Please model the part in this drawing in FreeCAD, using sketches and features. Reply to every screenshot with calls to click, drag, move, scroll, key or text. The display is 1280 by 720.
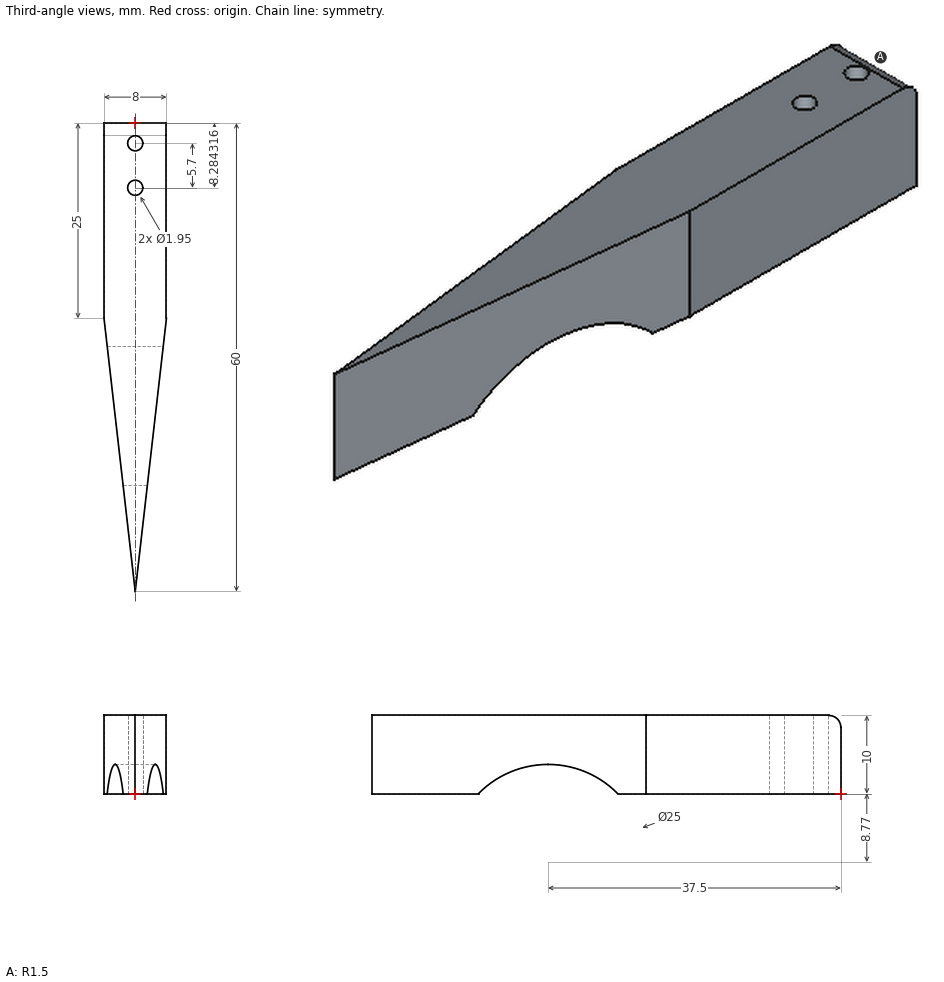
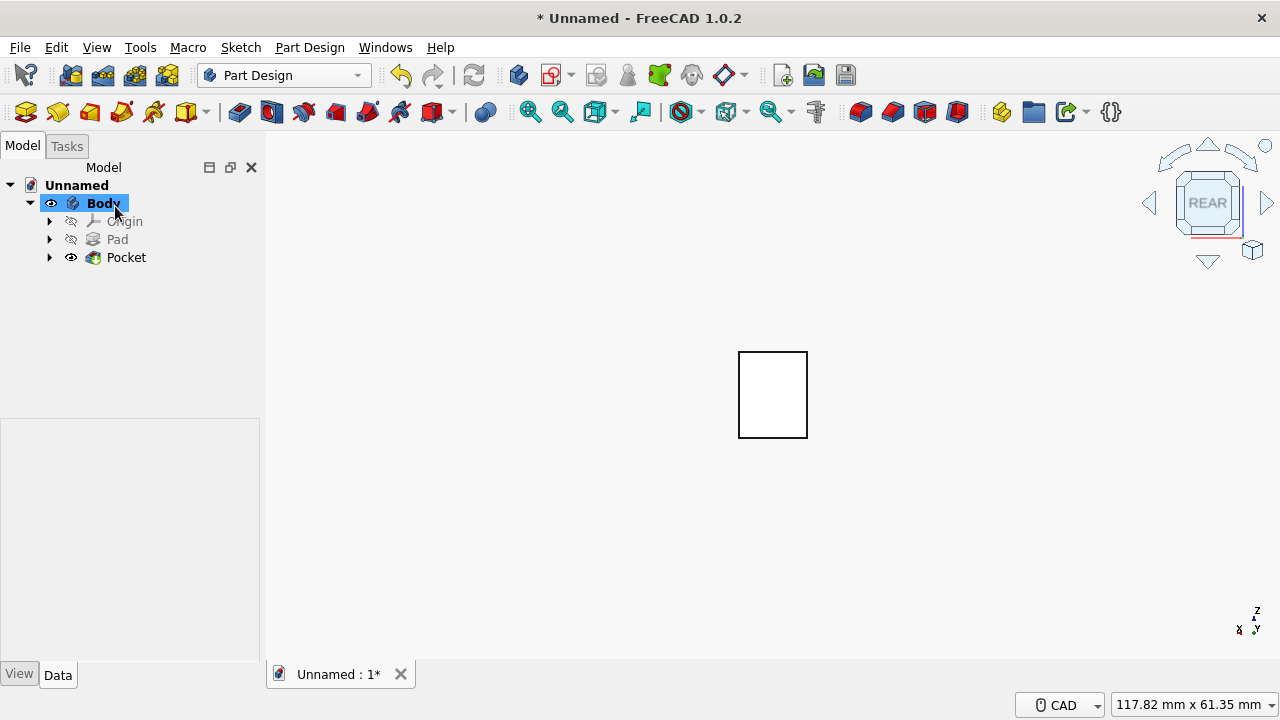
click(532, 112)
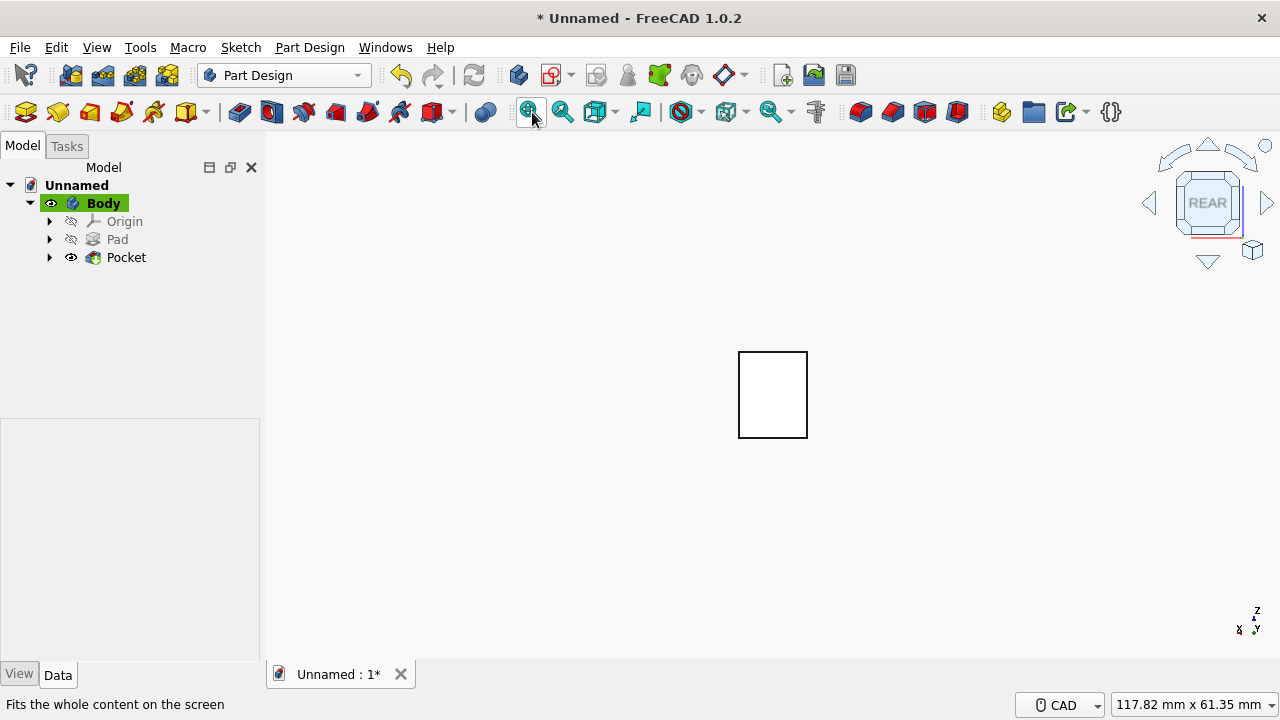
click(773, 351)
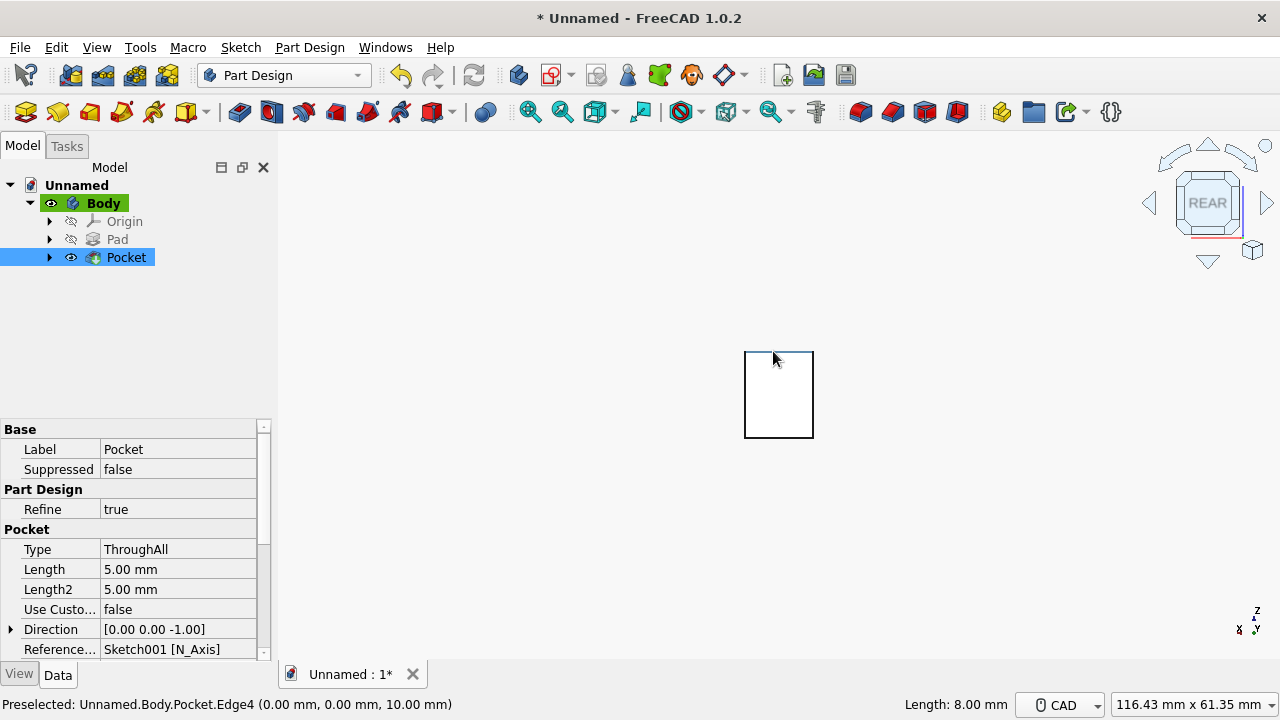
click(862, 112)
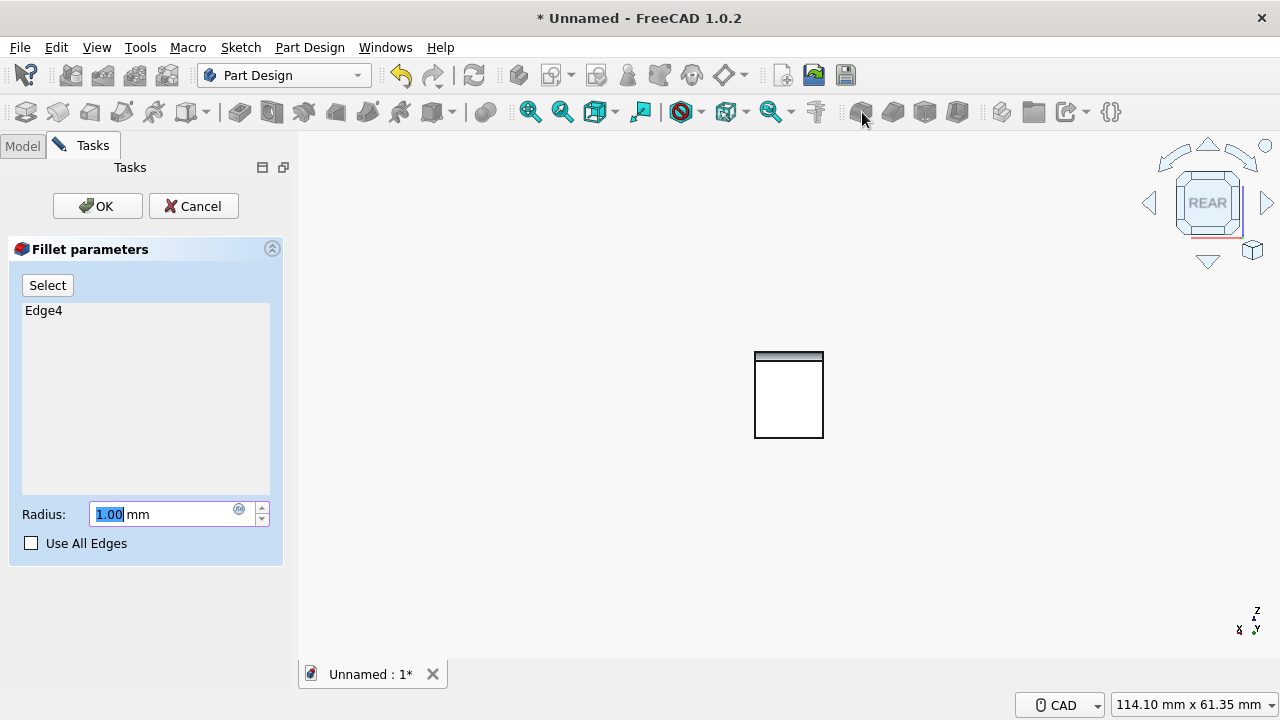
text(1.5)
key(Tab)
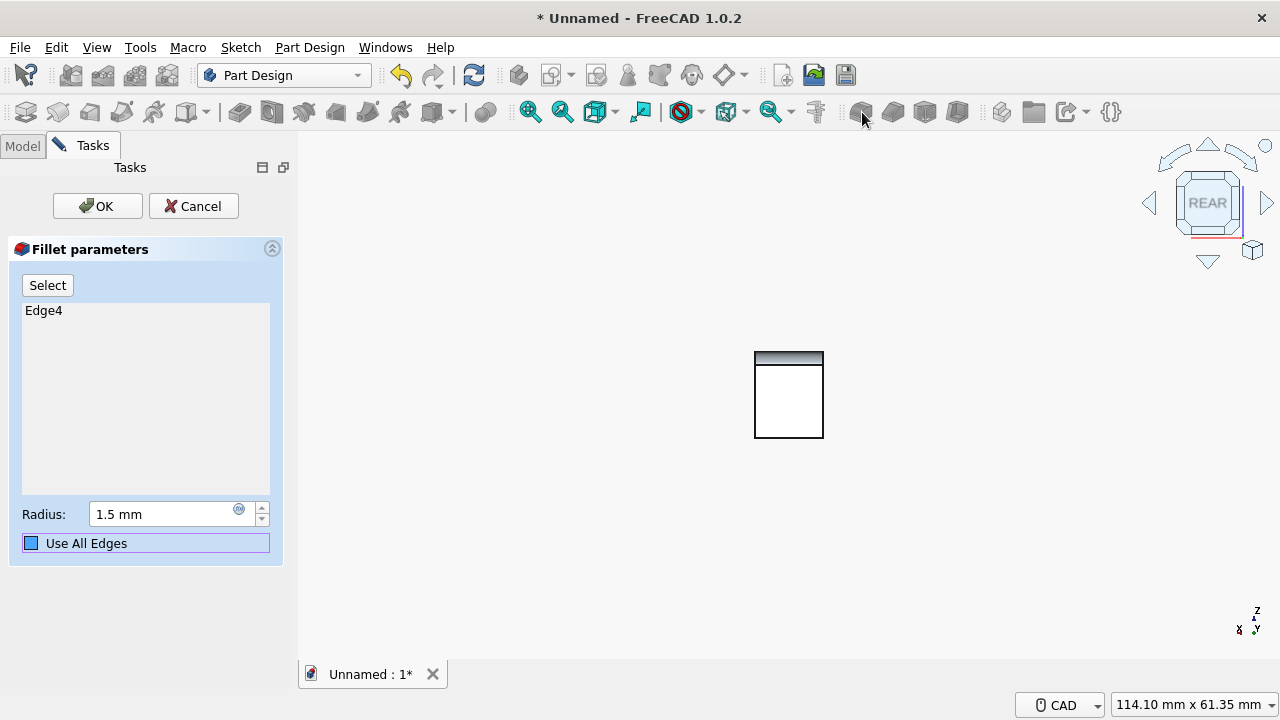
click(98, 206)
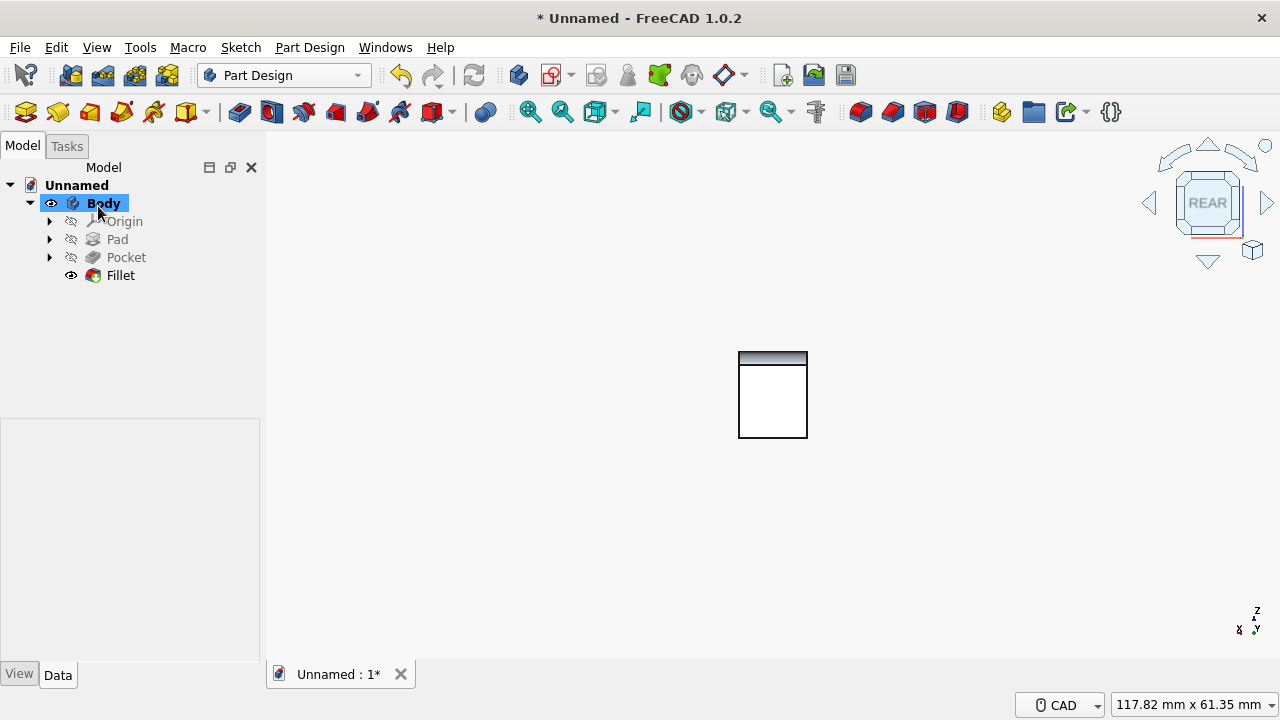
key(v)
key(f)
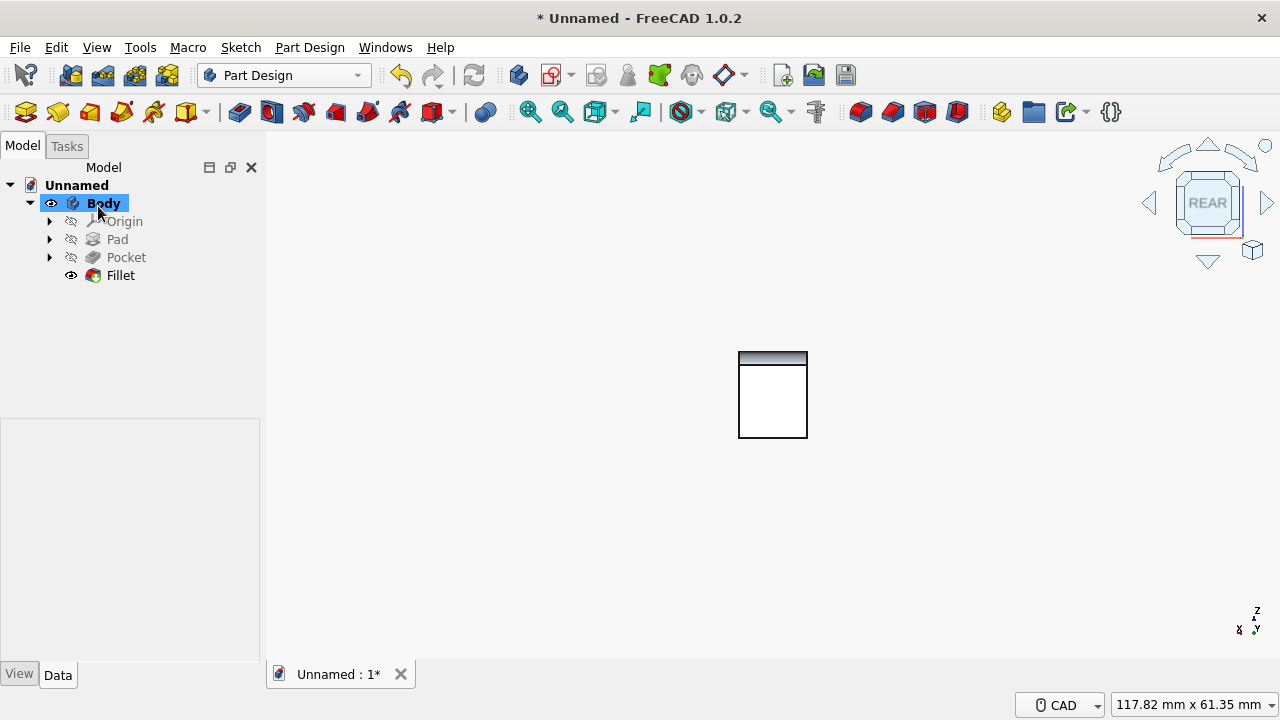
key(6)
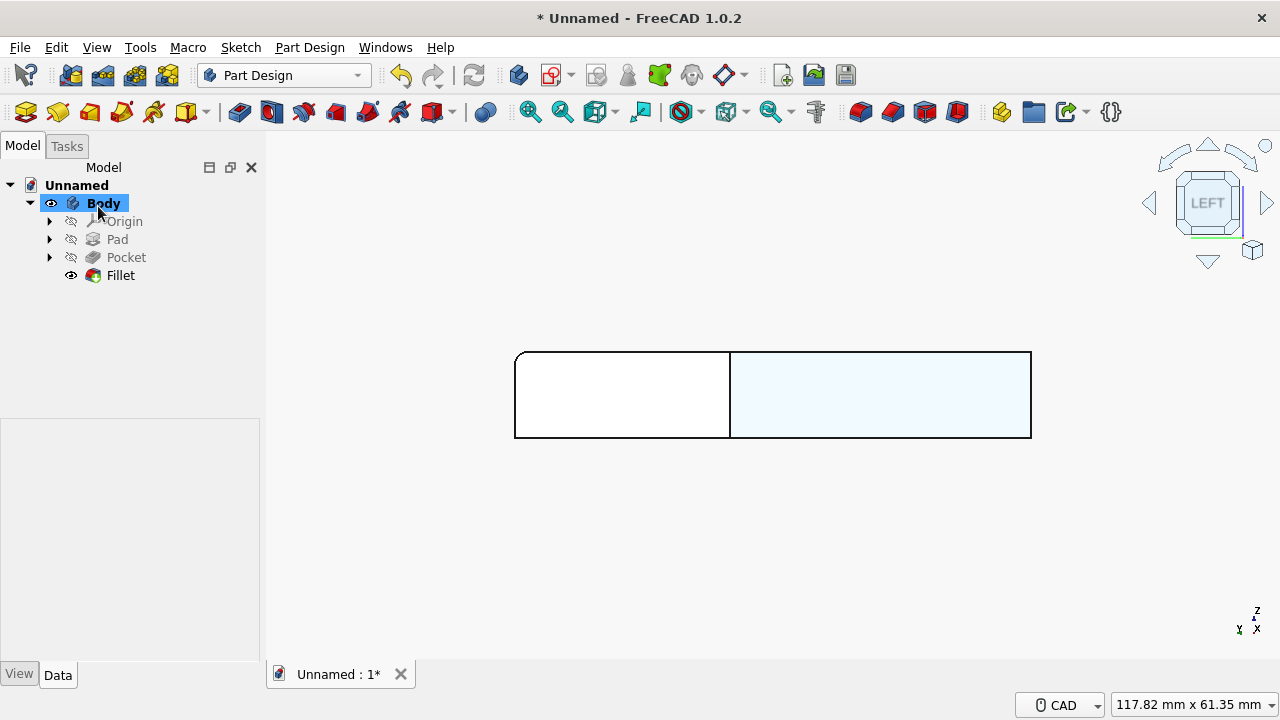
click(561, 394)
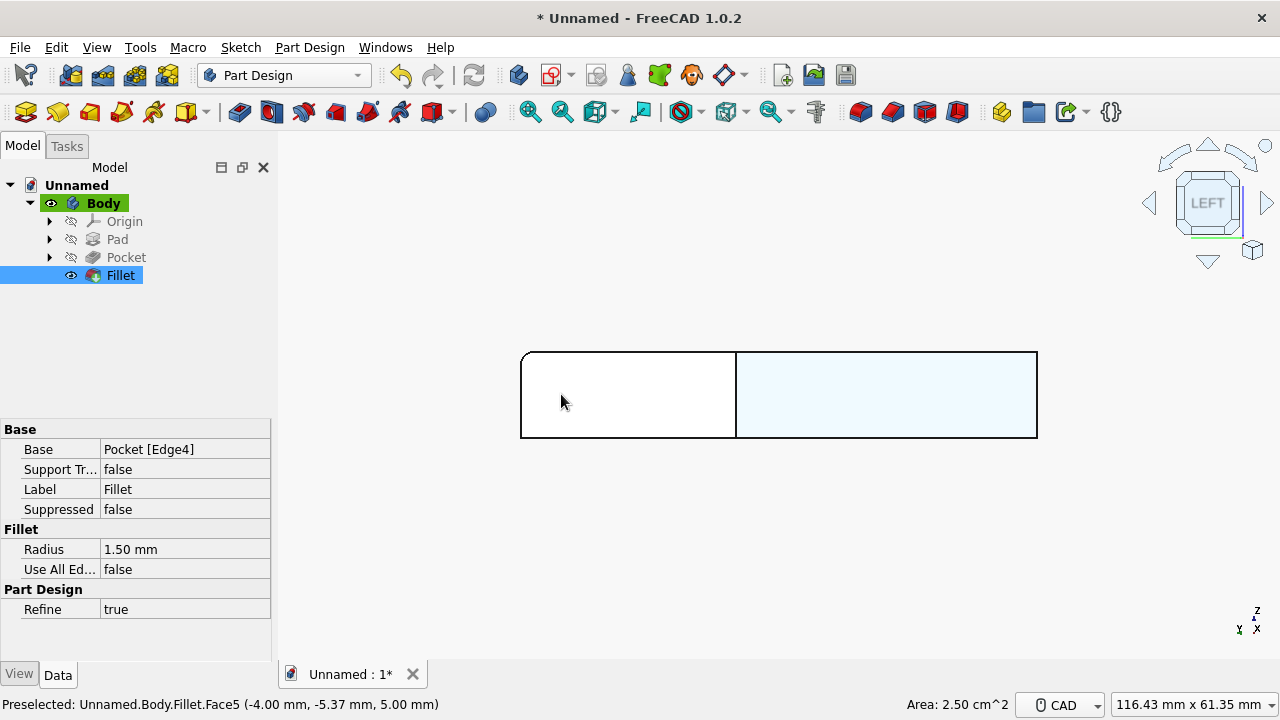
click(552, 76)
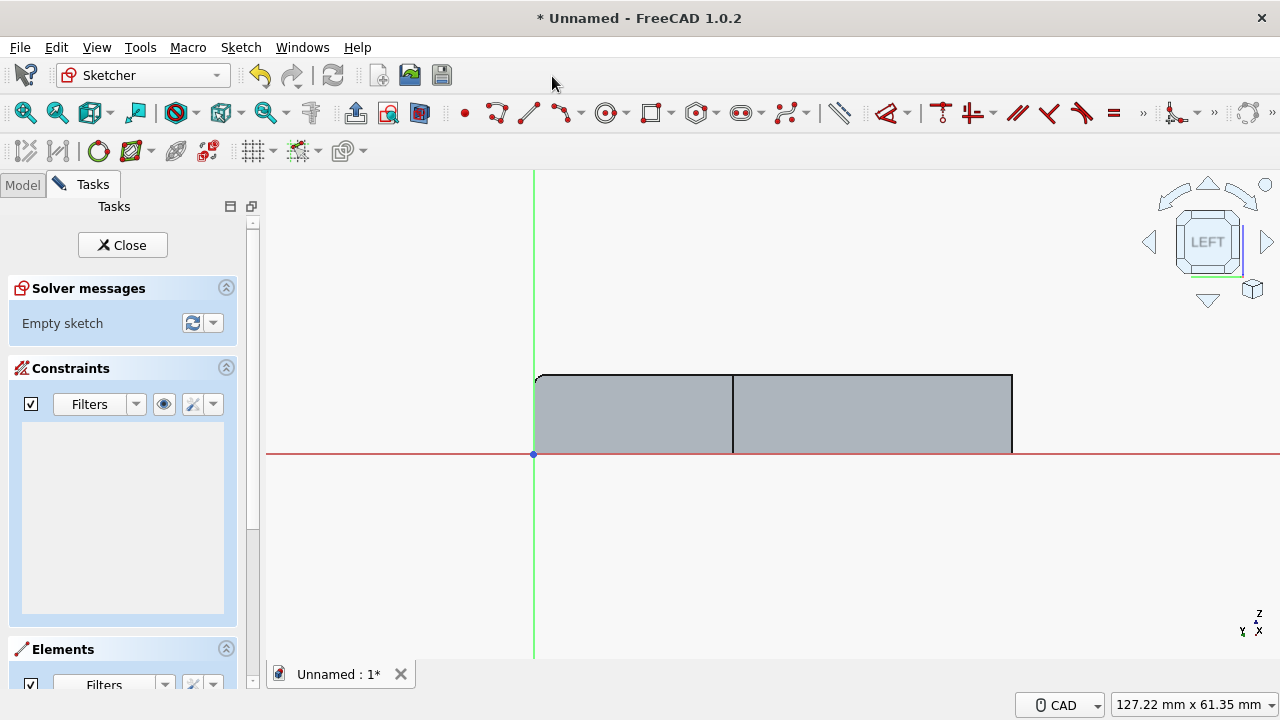
scroll(575, 198, down, 1)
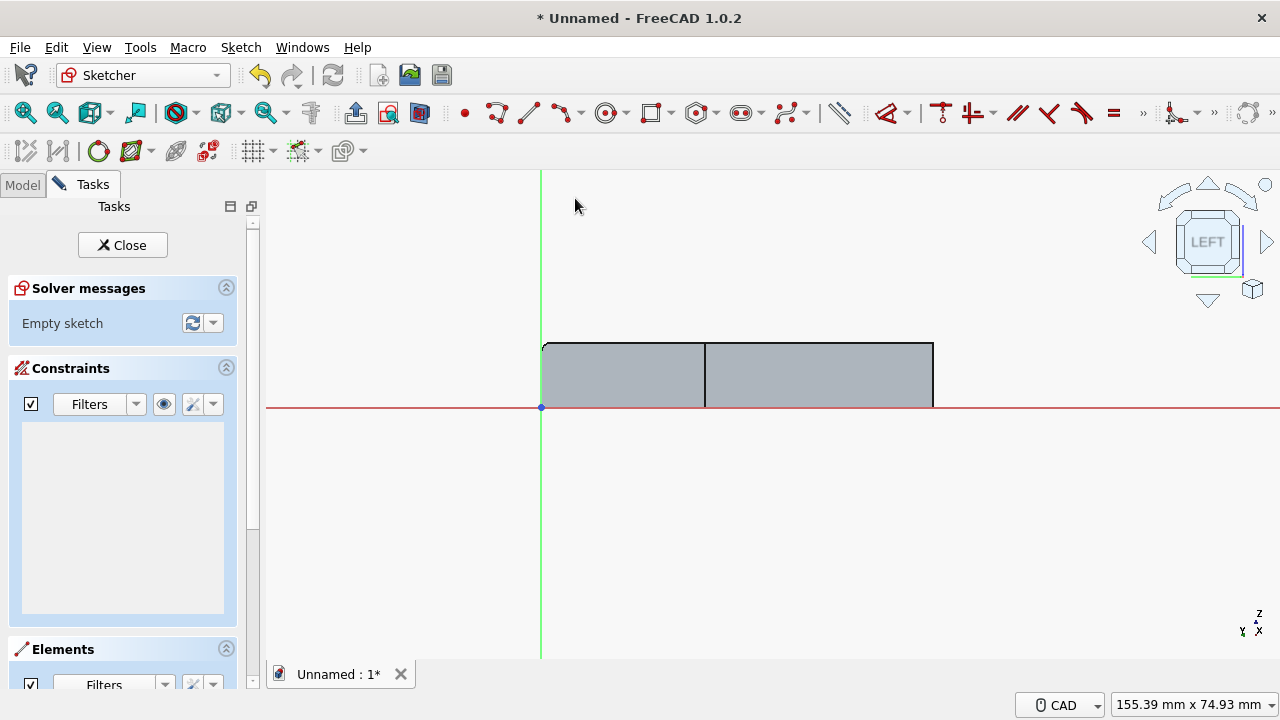
scroll(705, 527, up, 3)